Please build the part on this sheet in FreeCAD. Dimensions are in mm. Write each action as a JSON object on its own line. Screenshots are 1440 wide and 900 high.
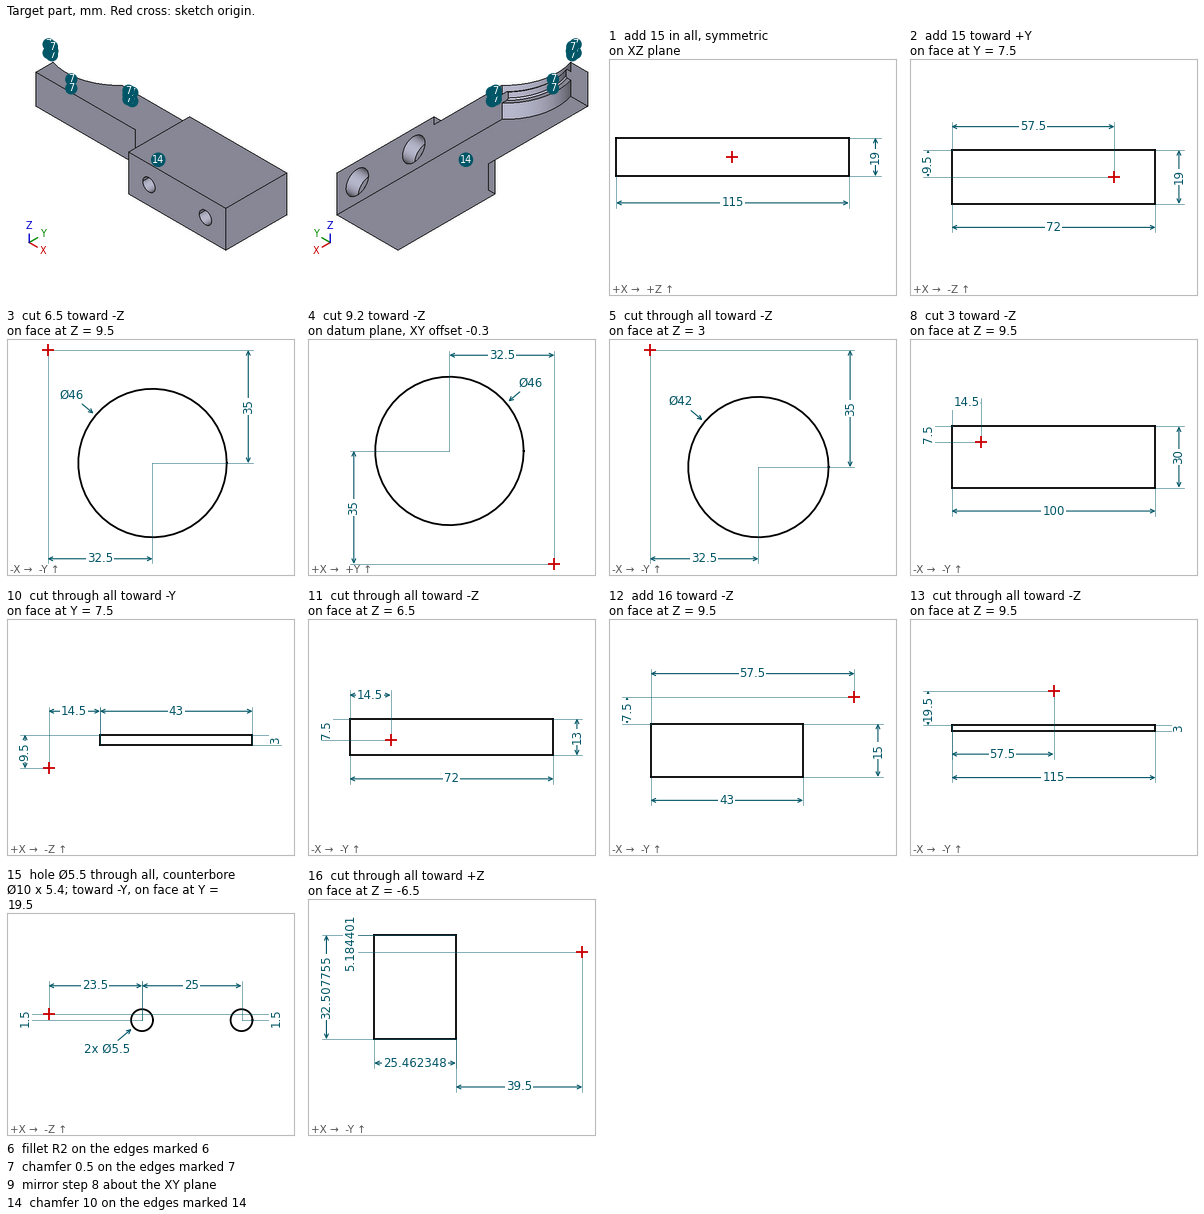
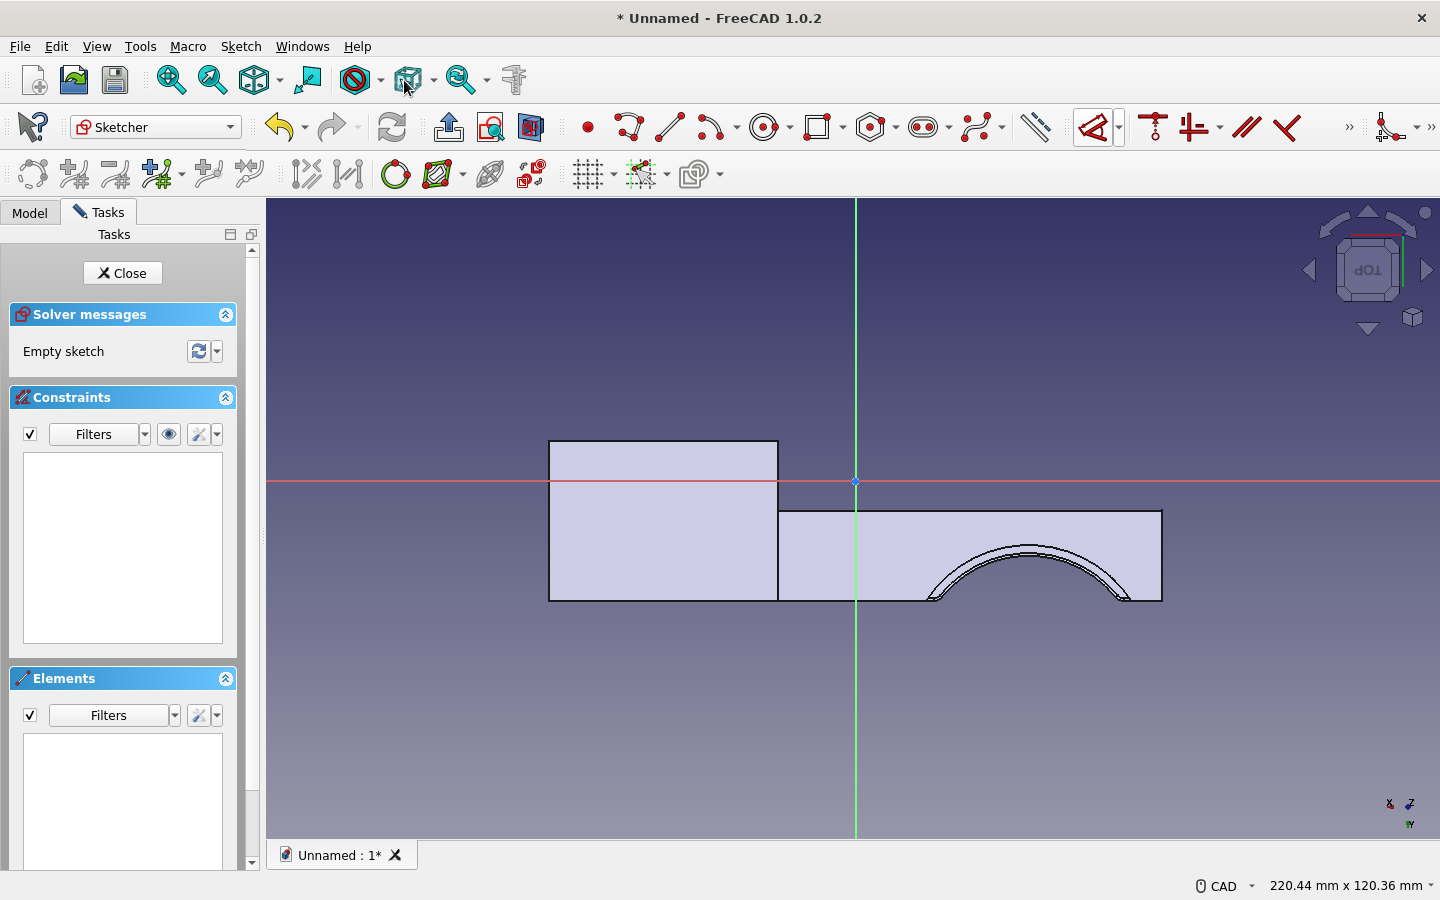
{"action": "left_click", "coordinate": [816, 128]}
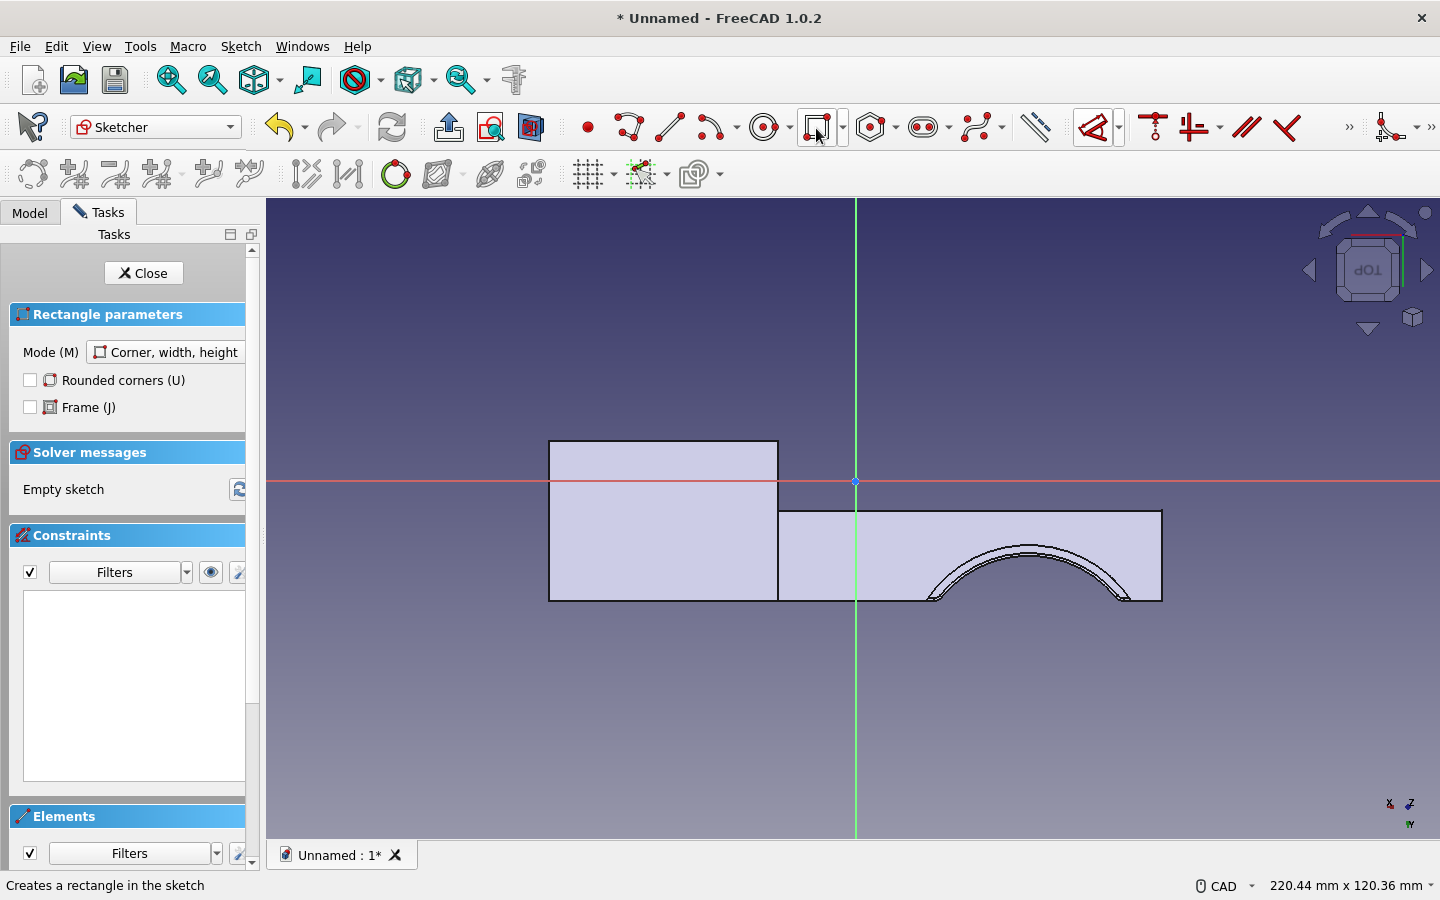
{"action": "left_click", "coordinate": [549, 585]}
{"action": "mouse_move", "coordinate": [1162, 601]}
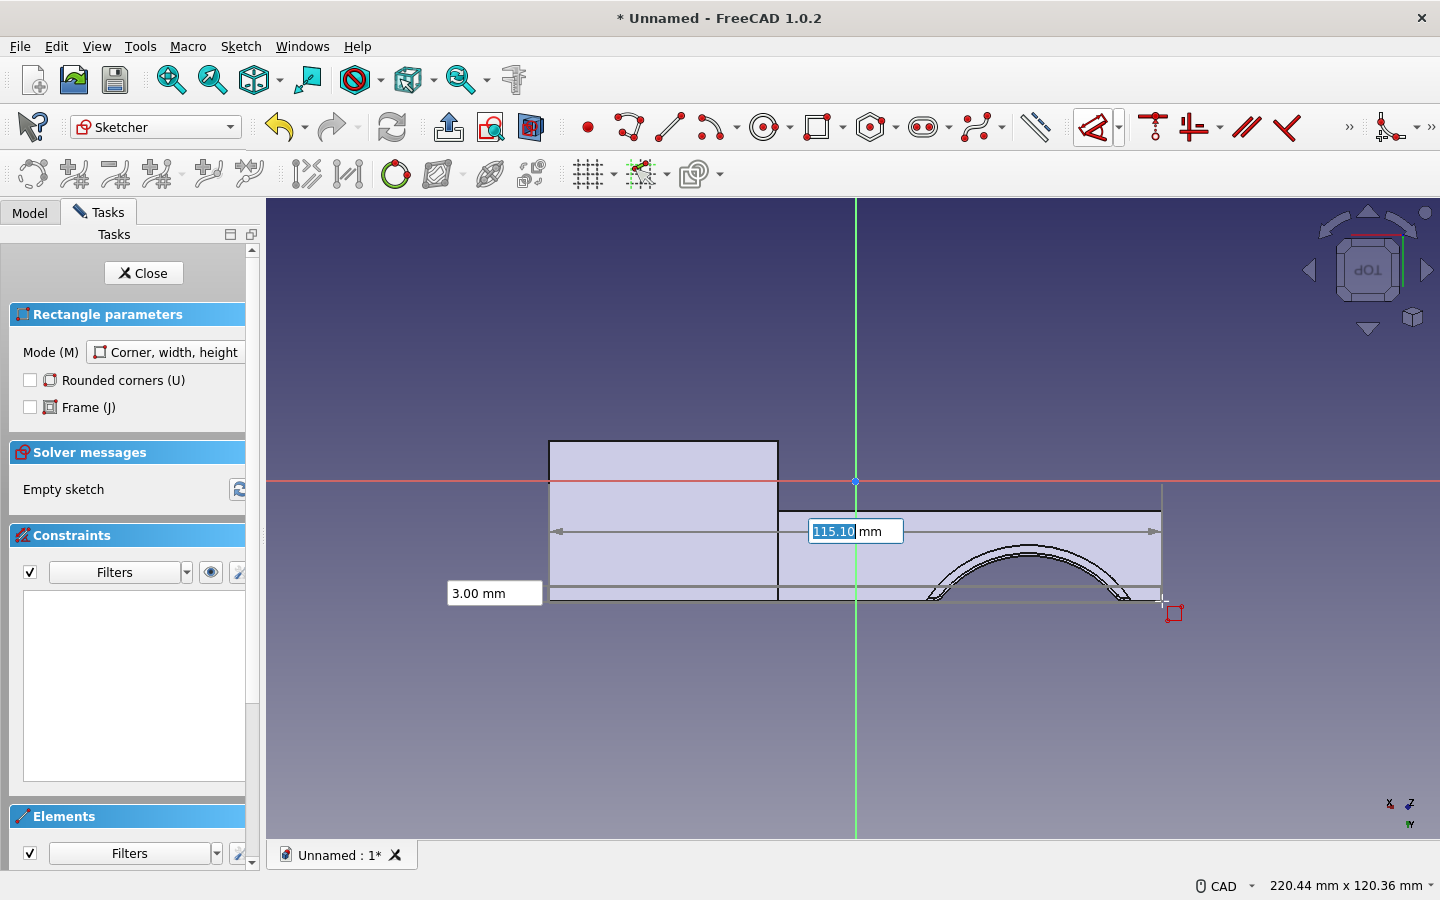
{"action": "type", "text": "115"}
{"action": "key", "text": "Tab"}
{"action": "type", "text": "3"}
{"action": "key", "text": "Return"}
{"action": "key", "text": "Escape"}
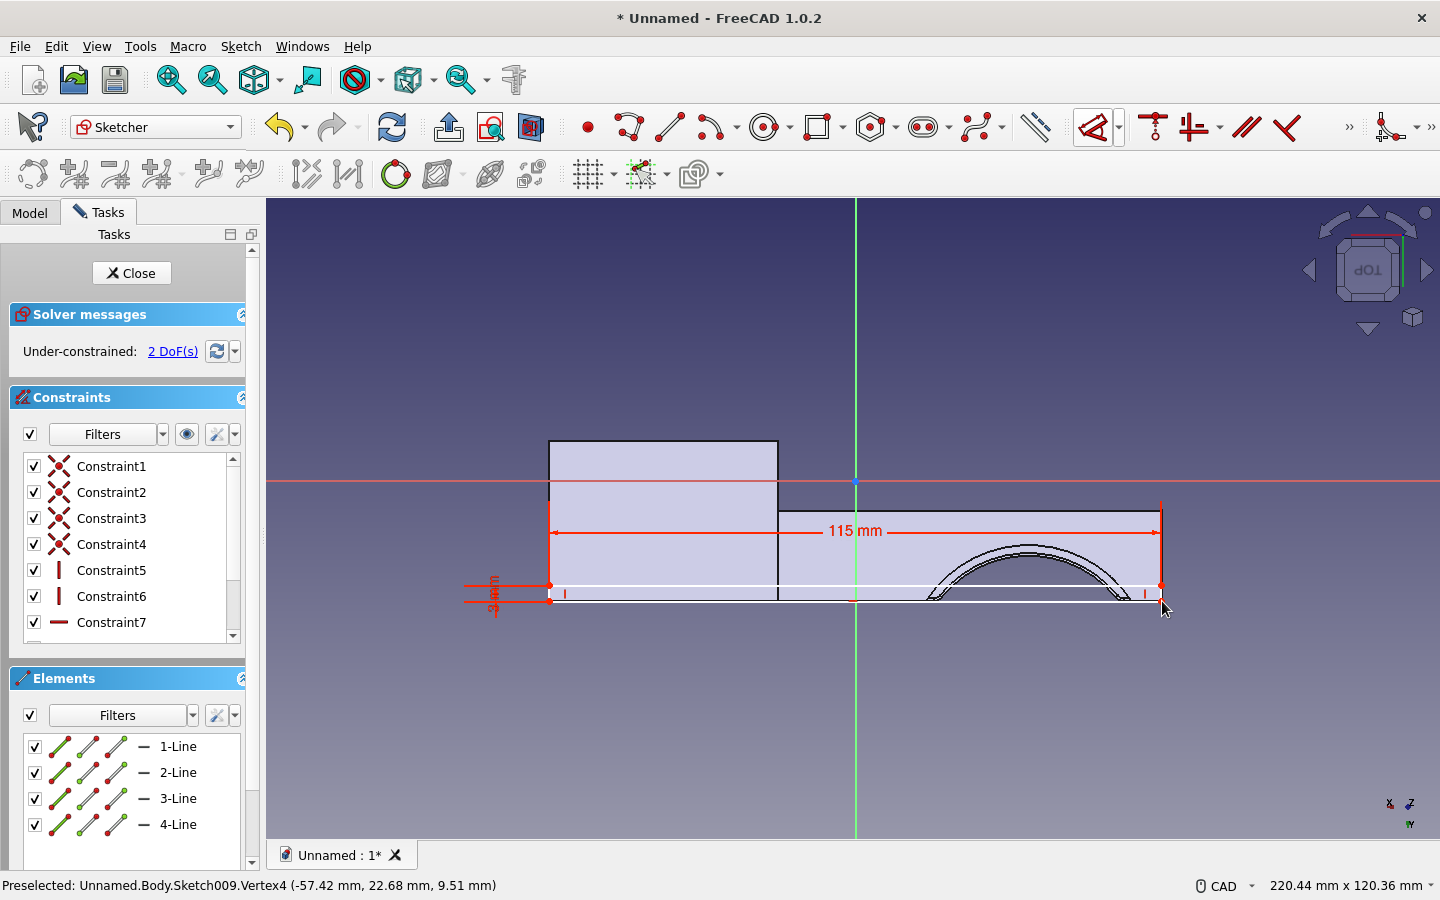
{"action": "left_click", "coordinate": [549, 586]}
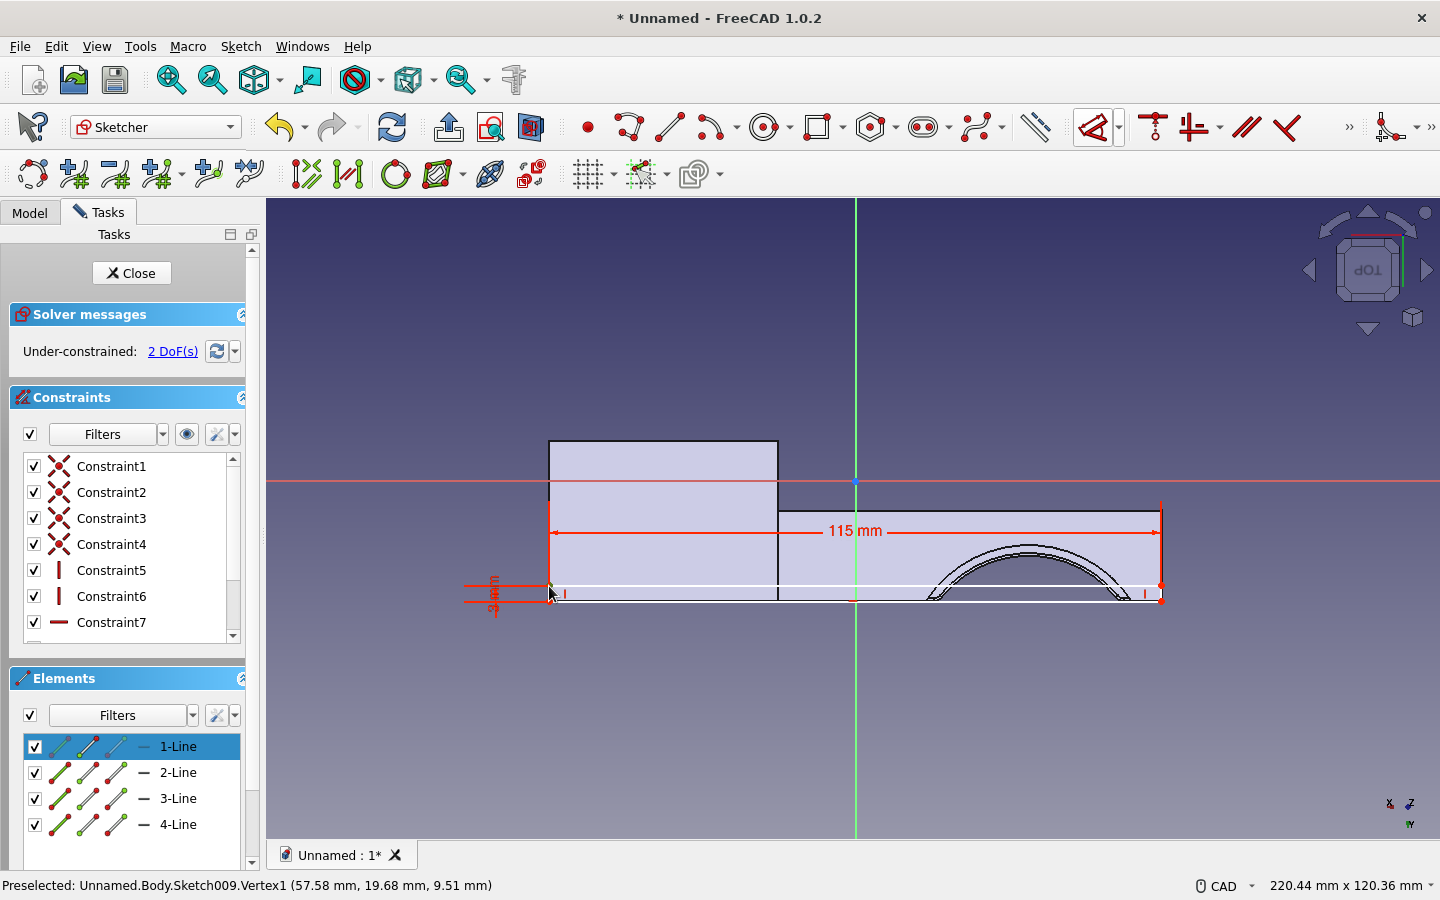
{"action": "key", "text": "l"}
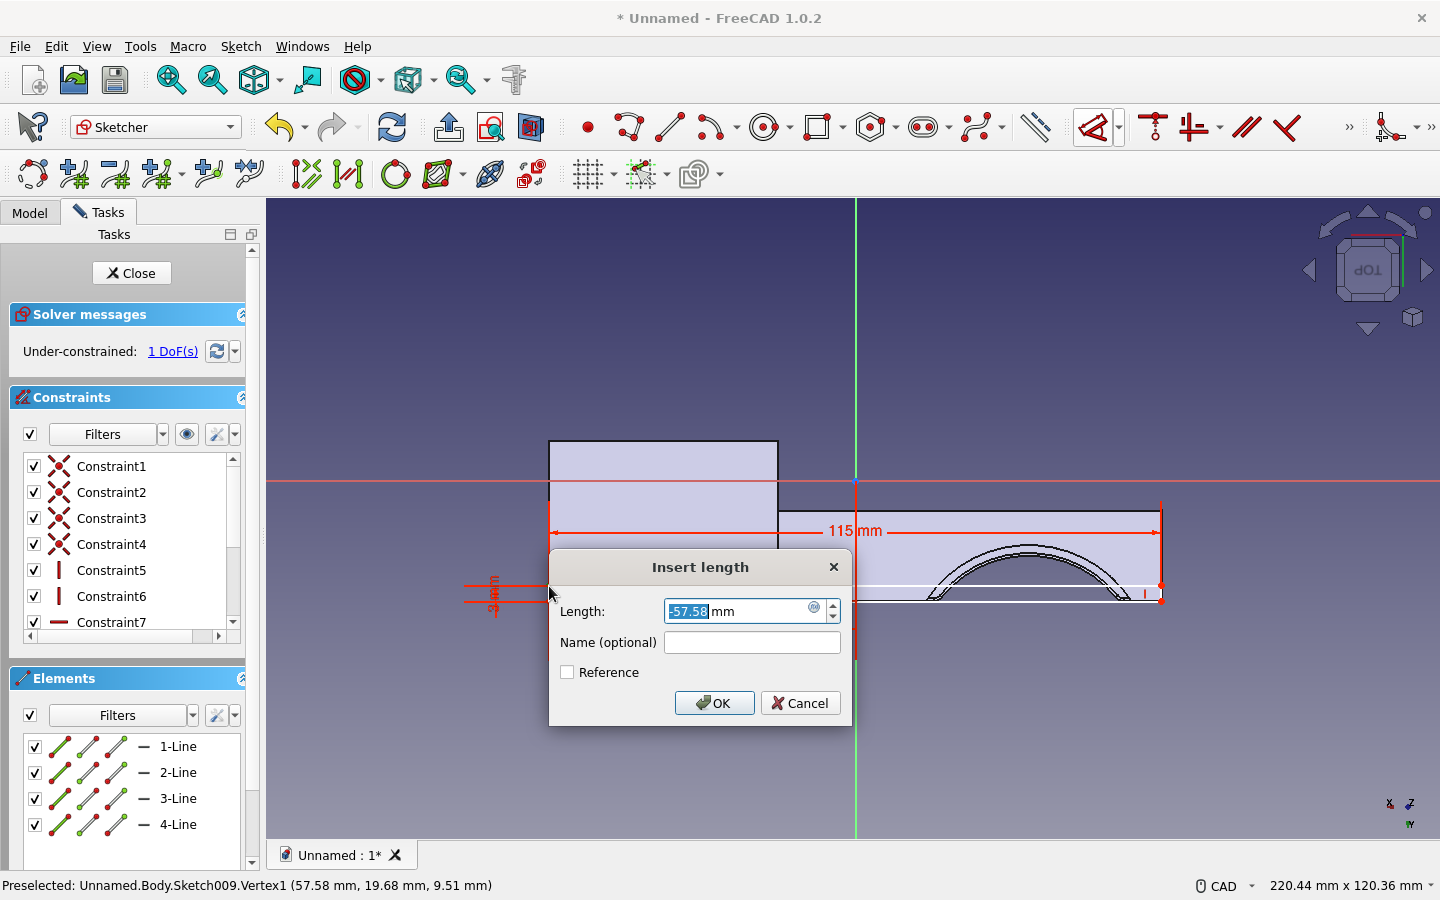
{"action": "type", "text": "-57.5"}
{"action": "key", "text": "Return"}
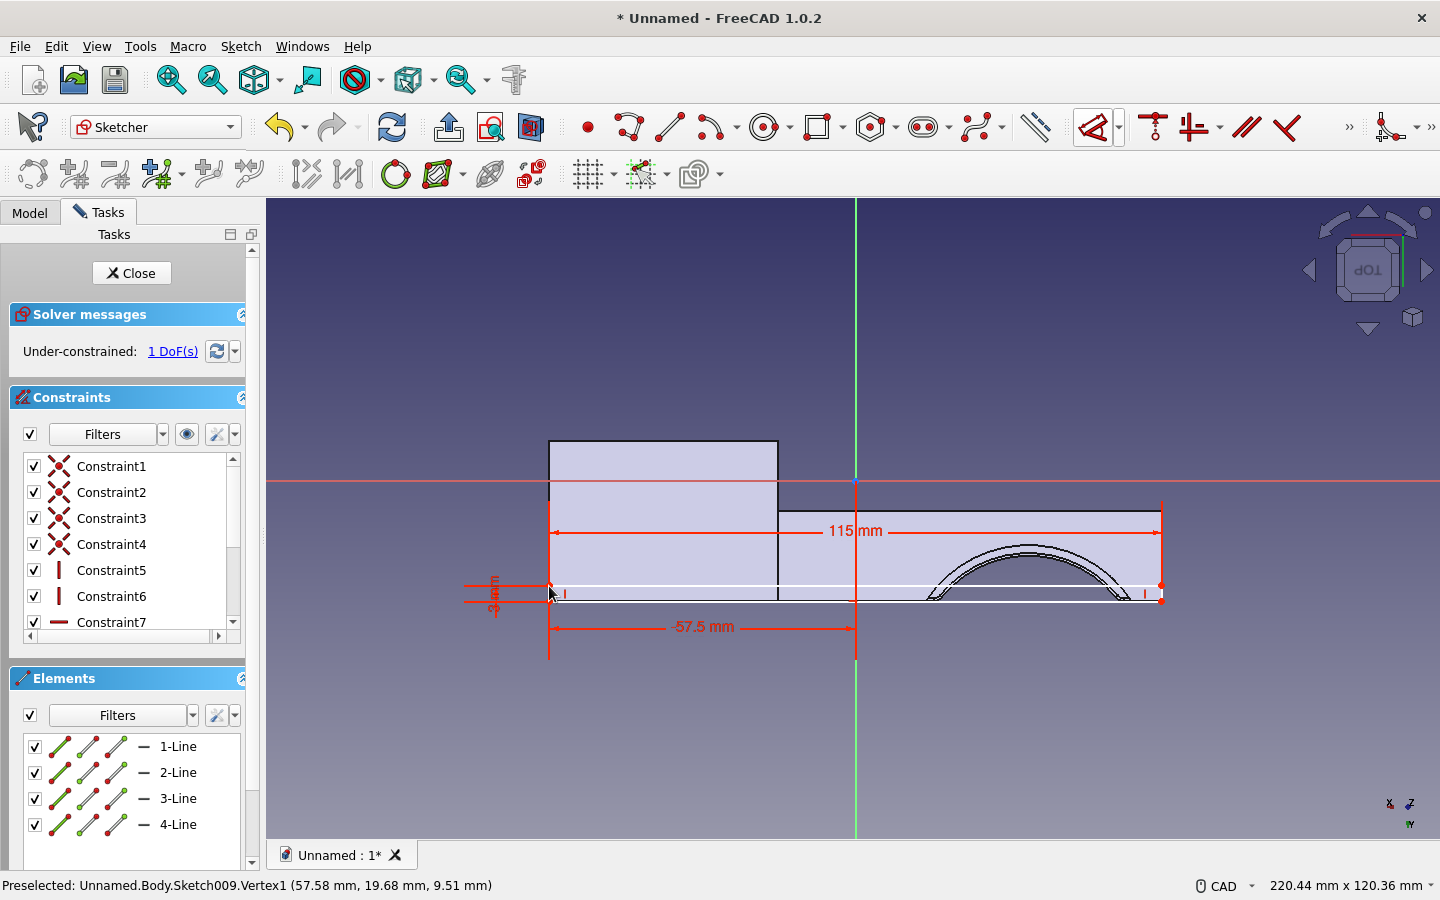
{"action": "left_click", "coordinate": [549, 586]}